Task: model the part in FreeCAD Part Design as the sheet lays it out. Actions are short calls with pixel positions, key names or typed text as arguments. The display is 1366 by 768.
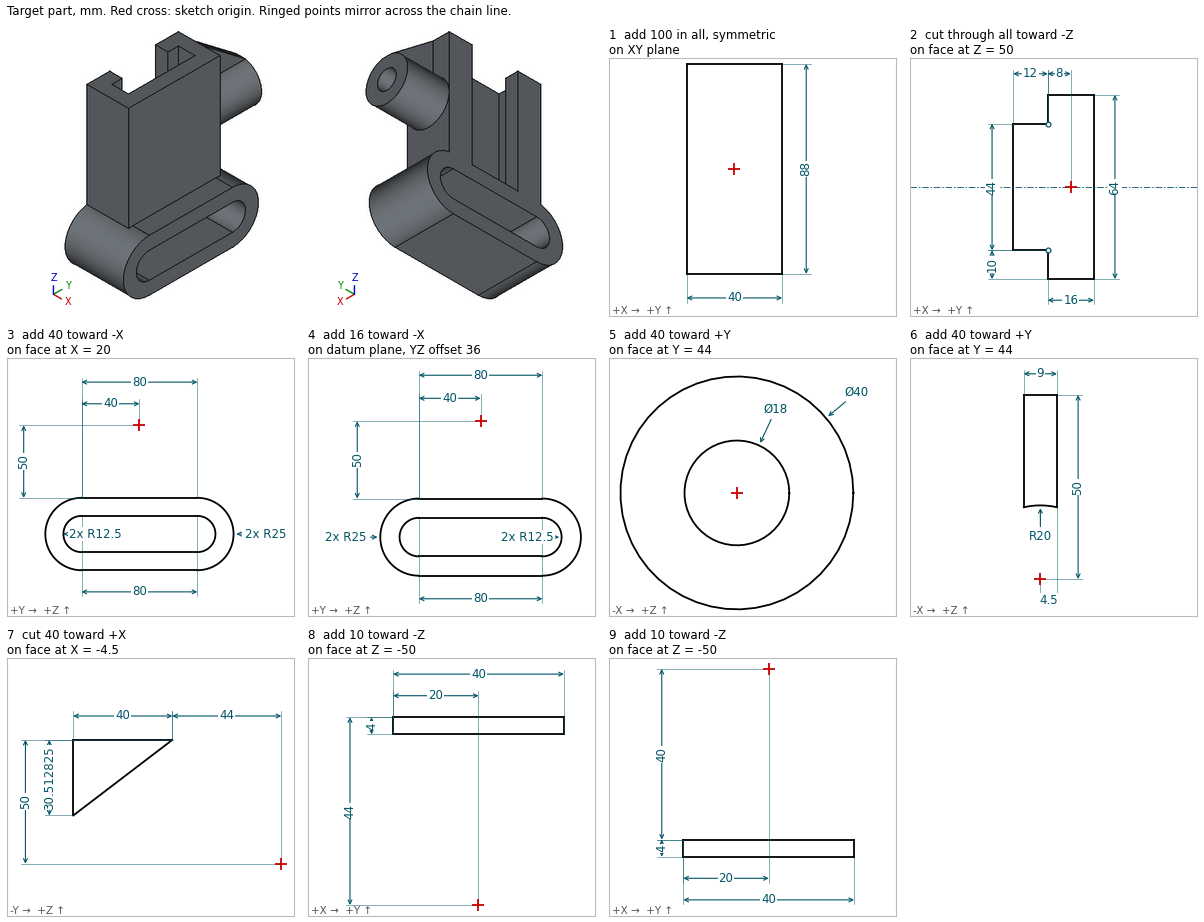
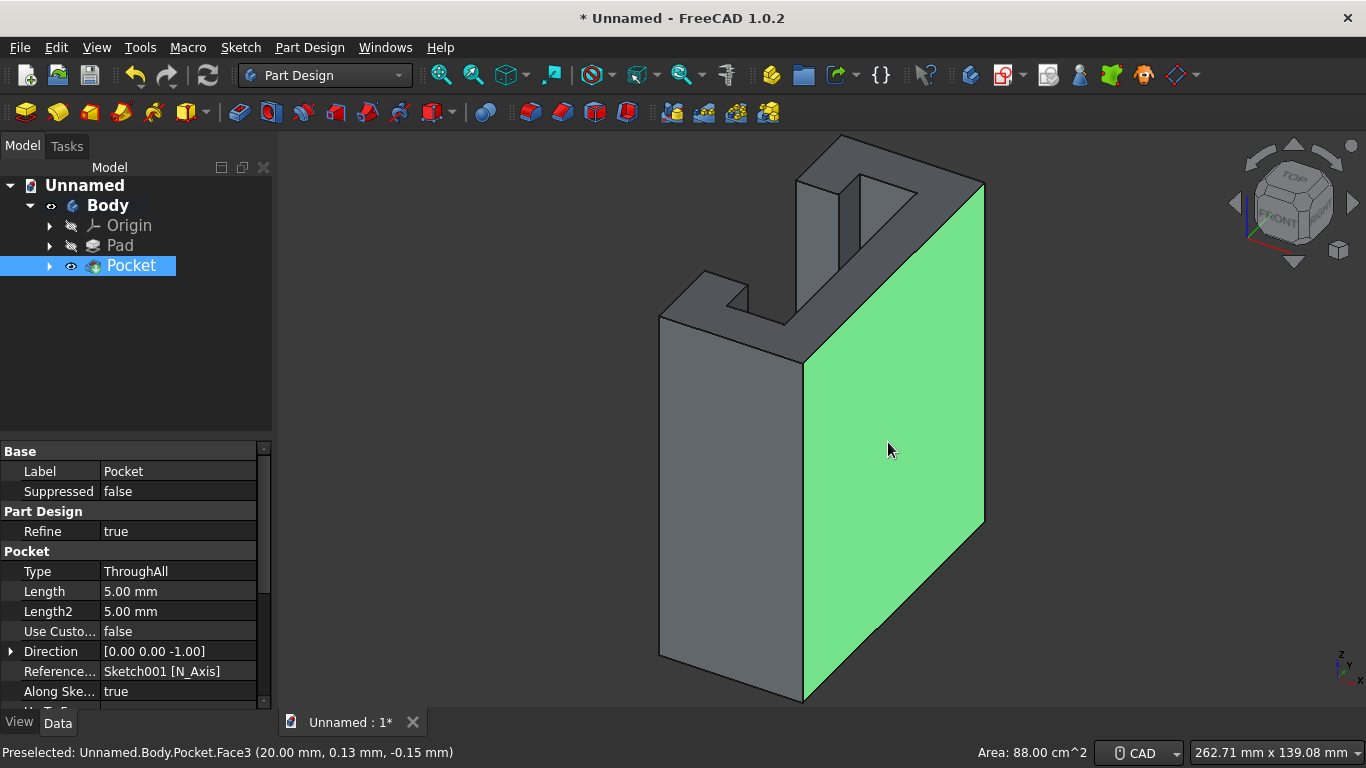
click(1004, 76)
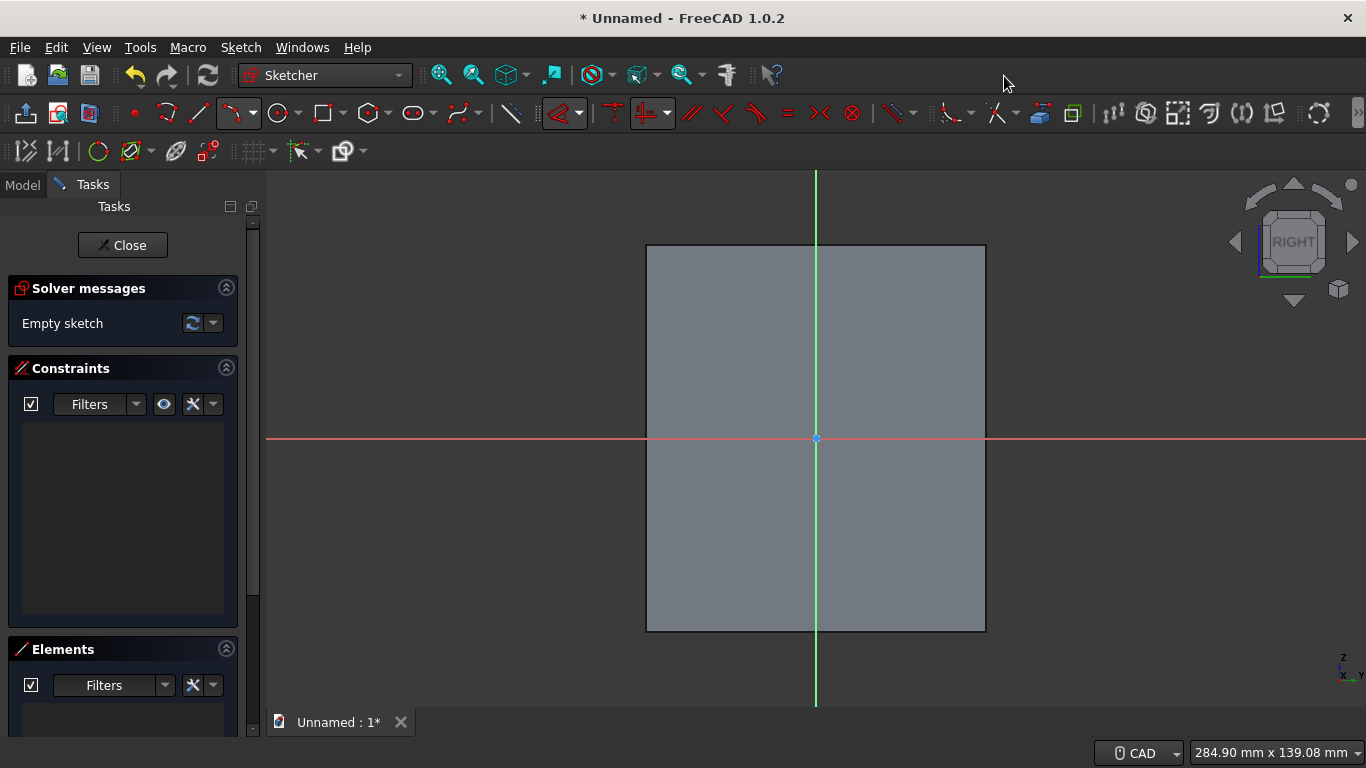
scroll(608, 198, down, 2)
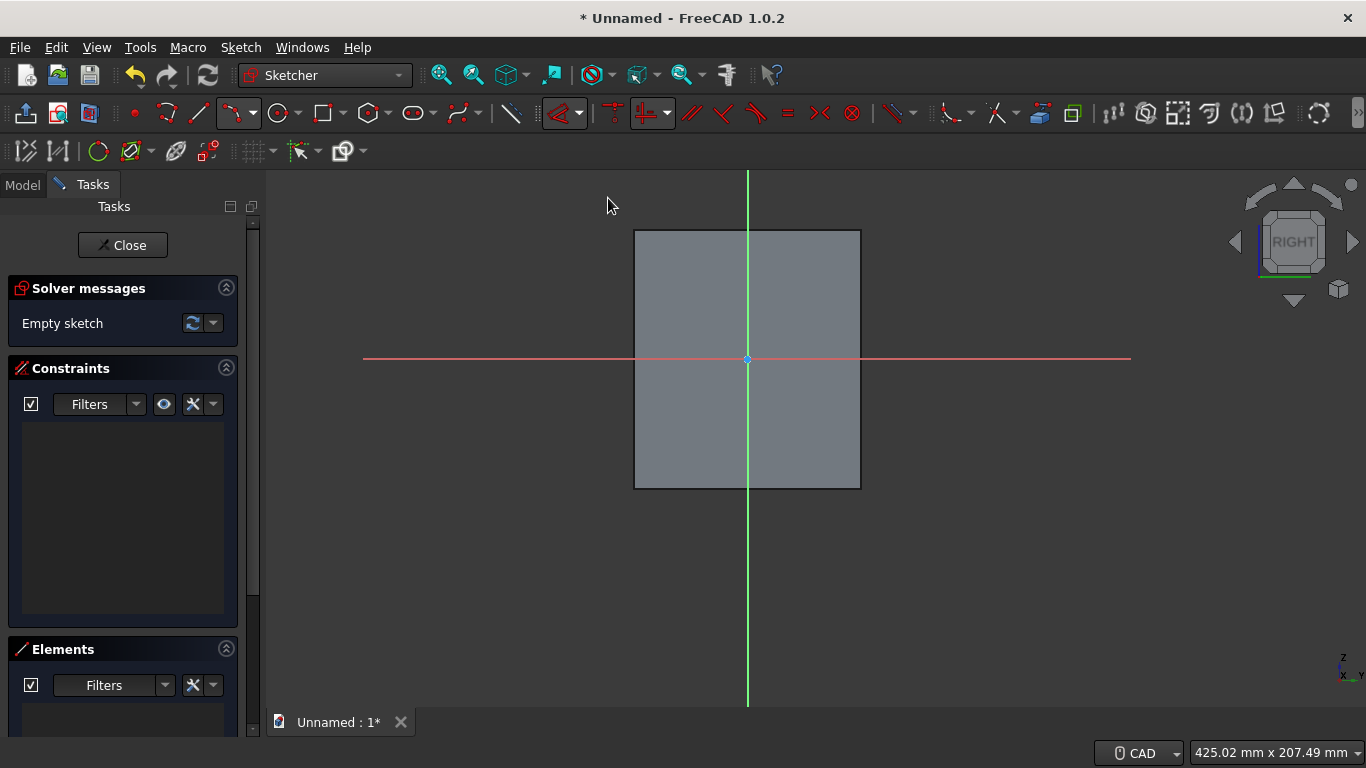
key(g)
key(s)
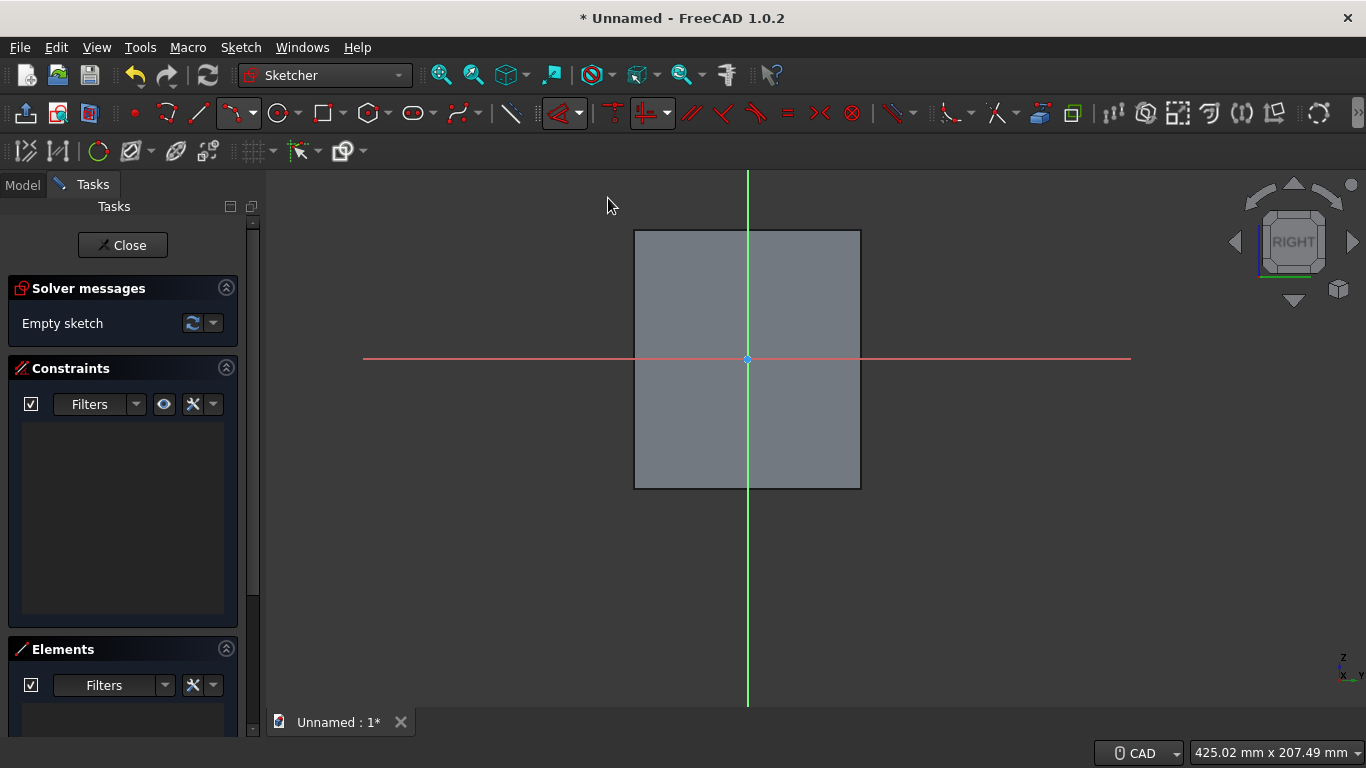
click(644, 553)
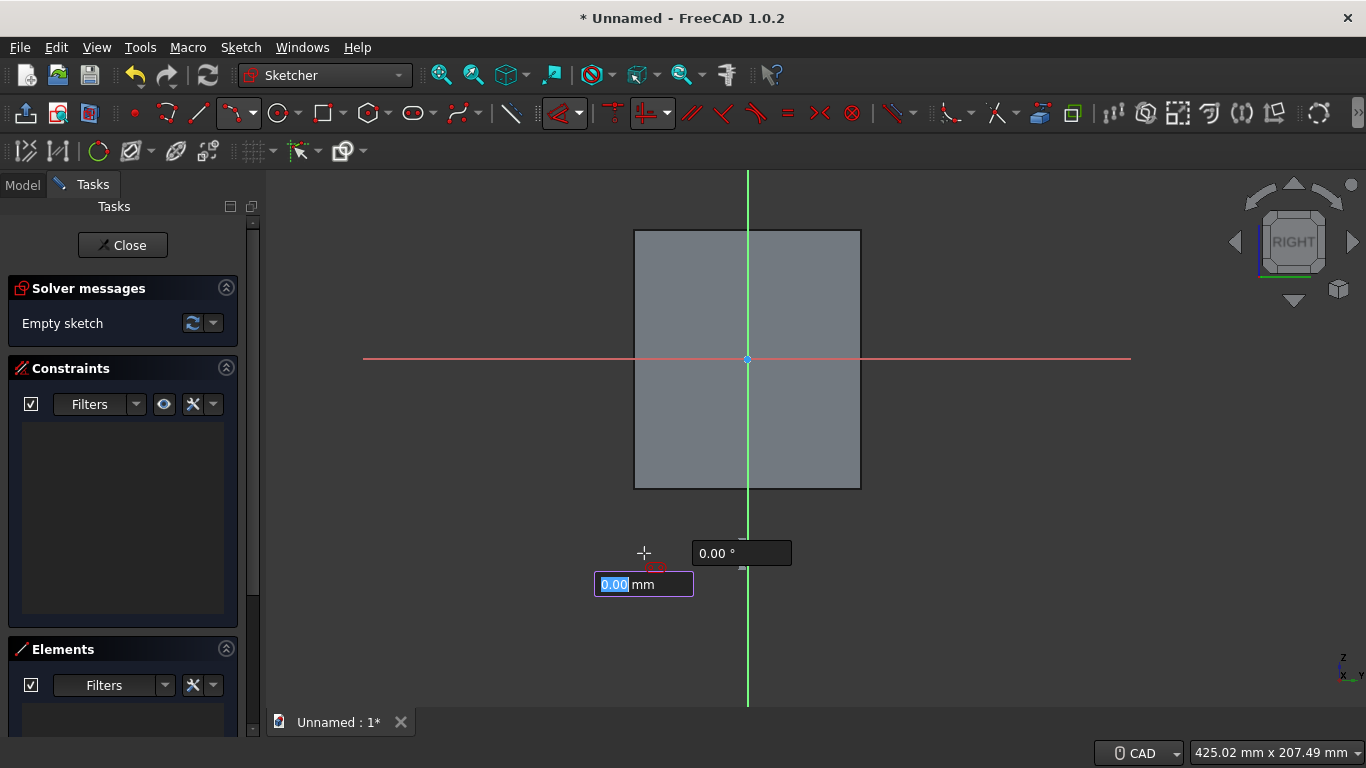
click(851, 553)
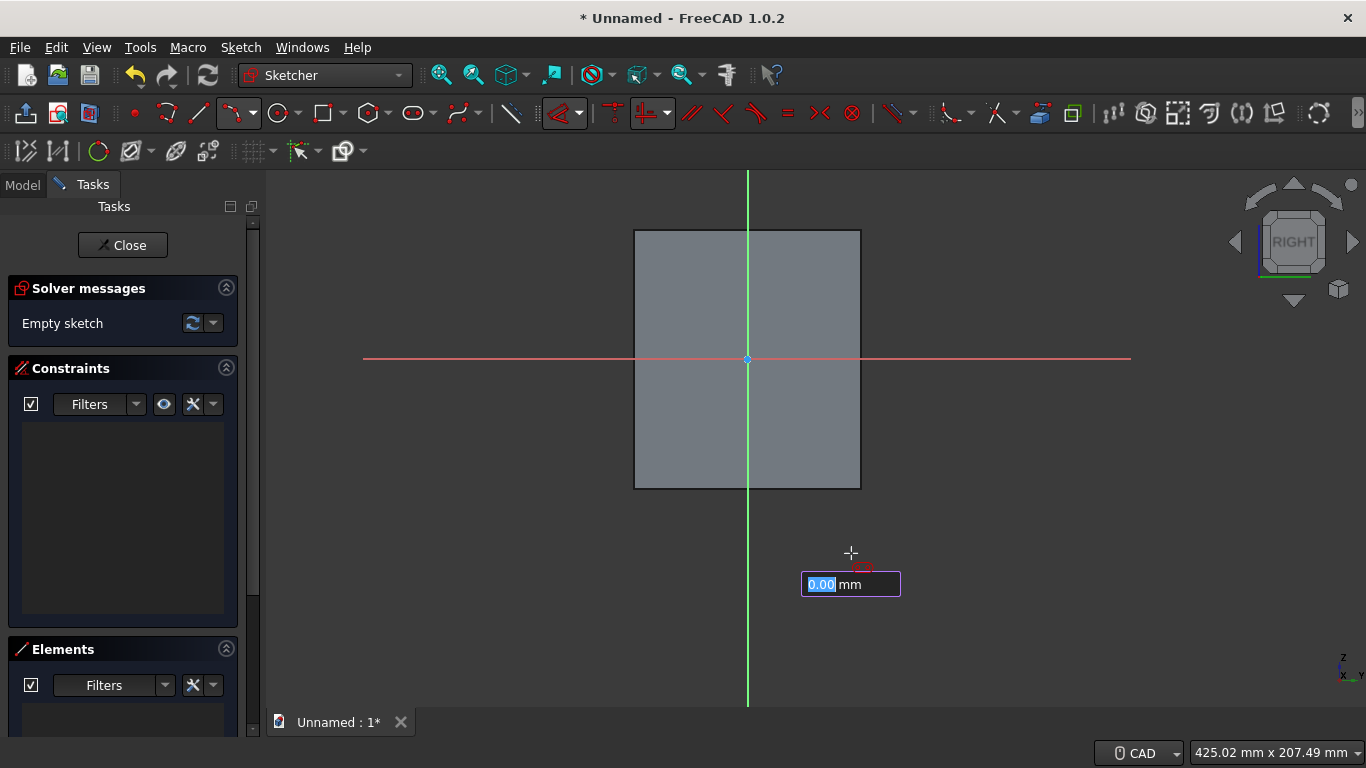
click(716, 618)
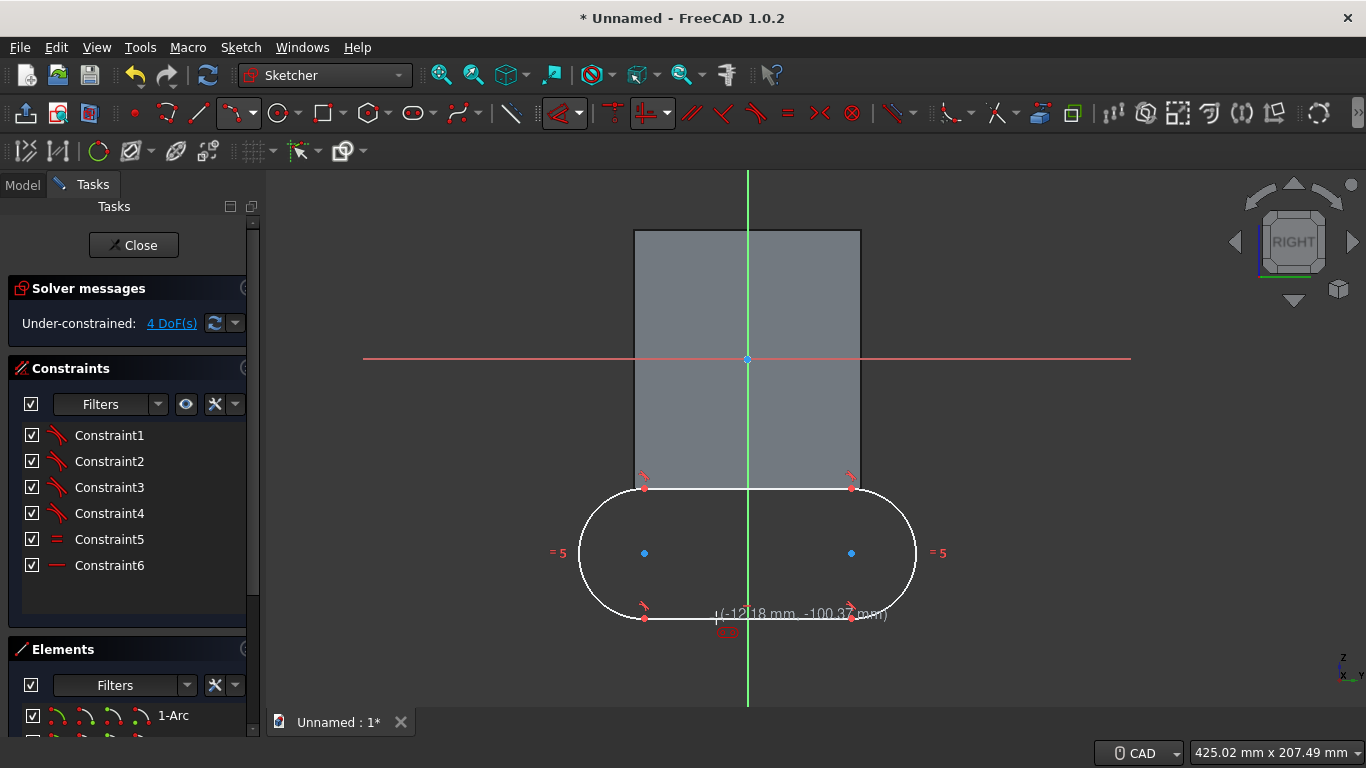
click(644, 554)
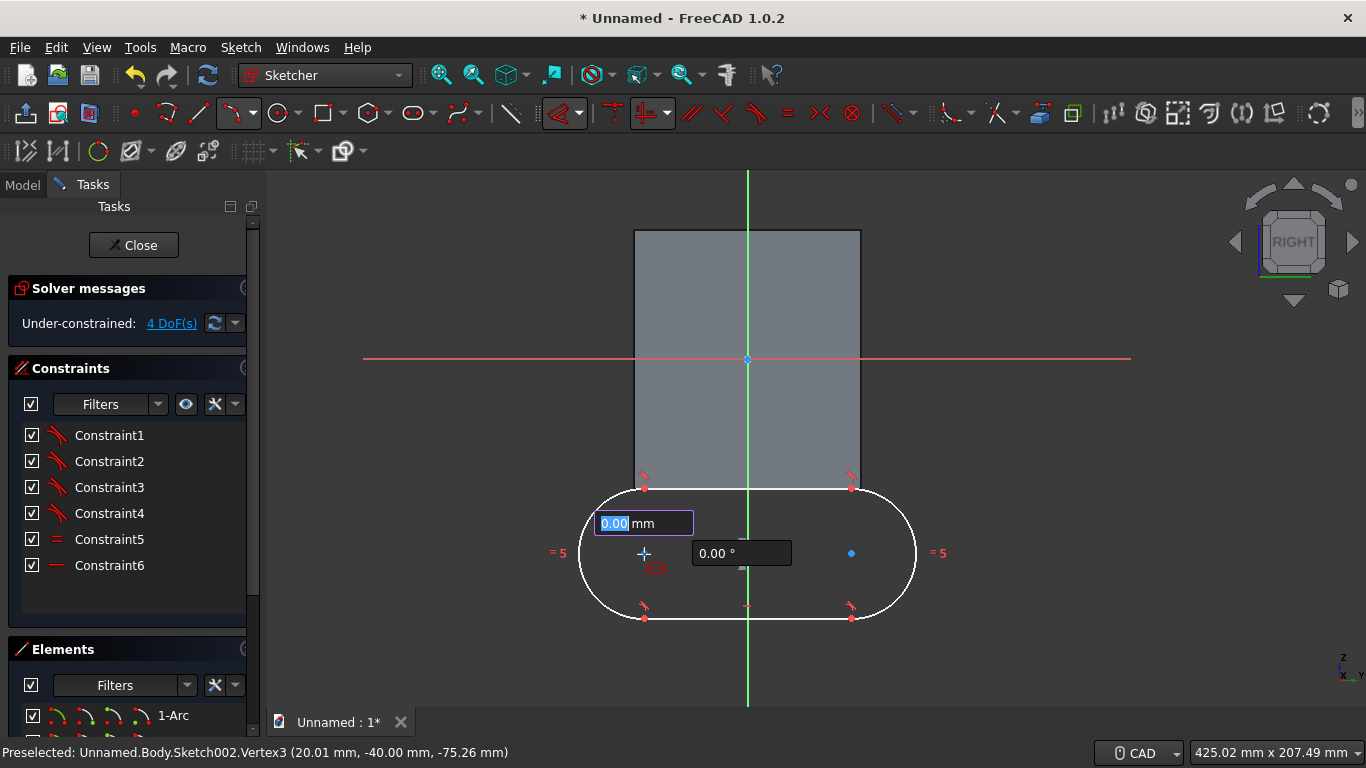
click(851, 554)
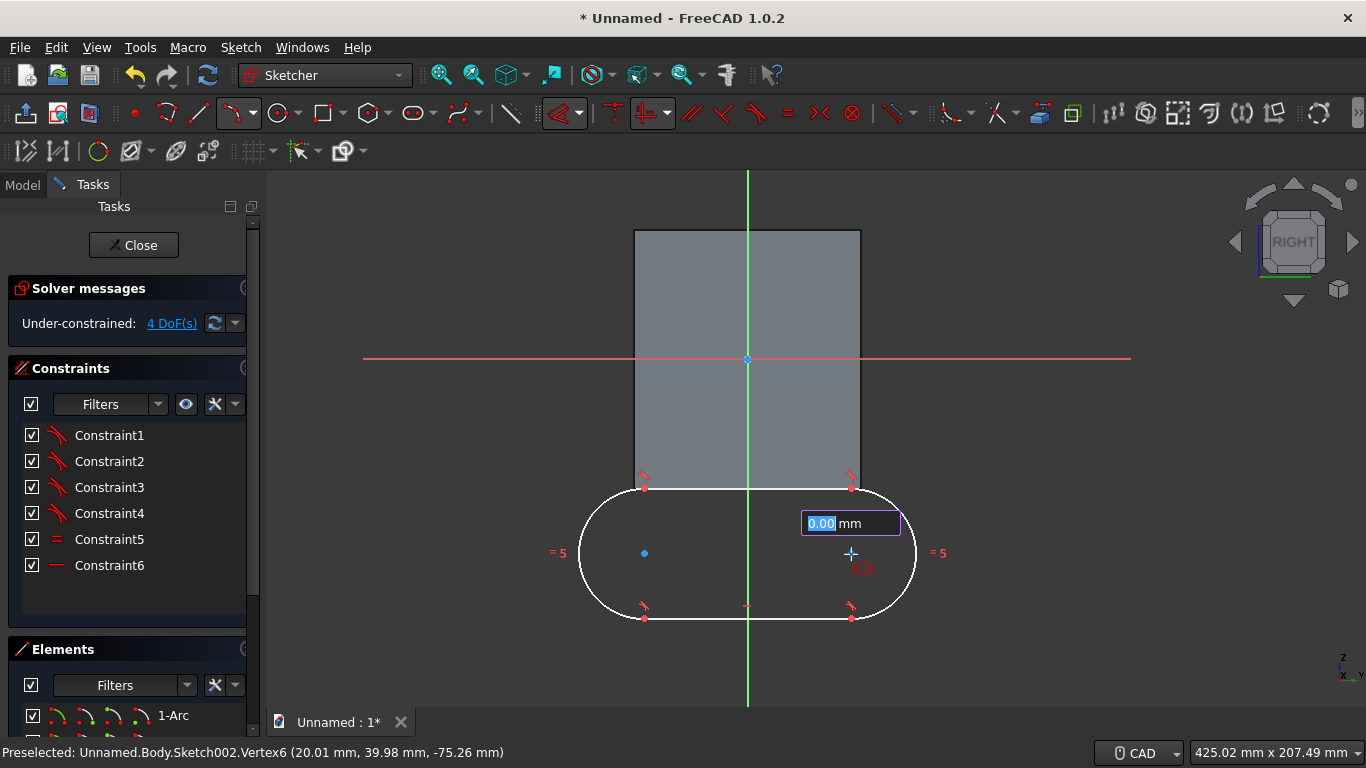
click(716, 521)
key(Escape)